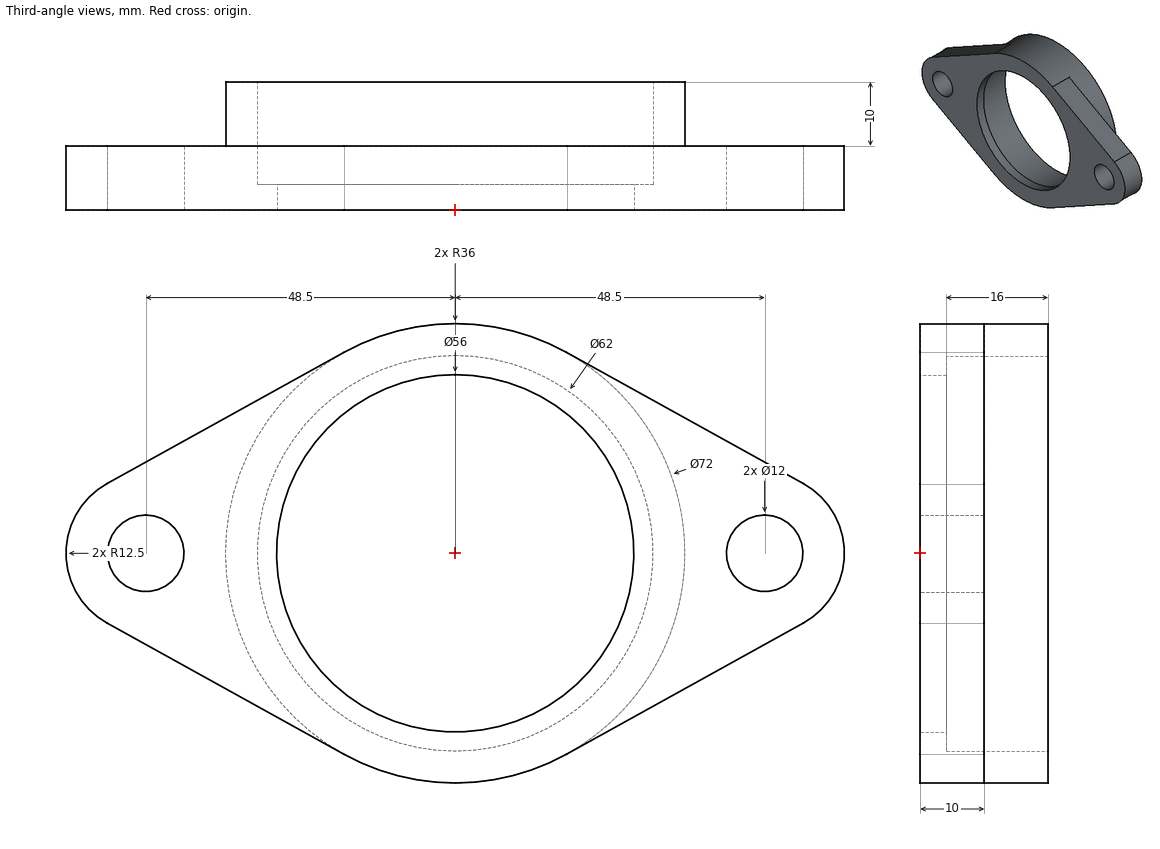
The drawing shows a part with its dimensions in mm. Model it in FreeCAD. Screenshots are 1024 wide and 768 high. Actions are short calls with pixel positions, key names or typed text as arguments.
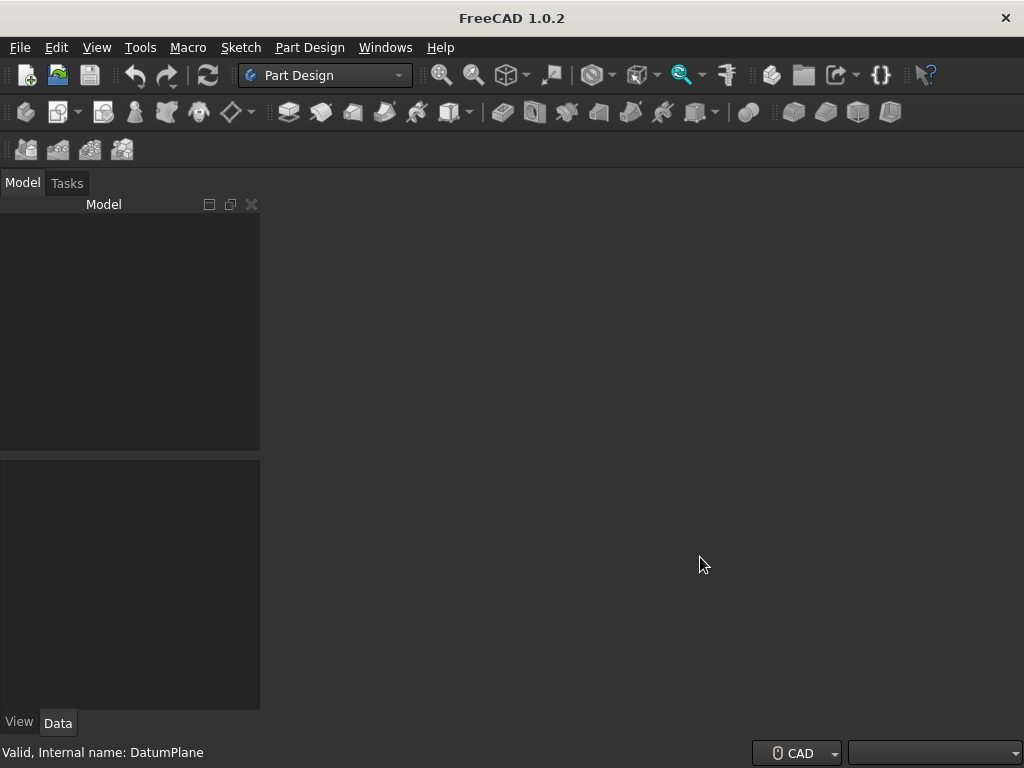
click(26, 76)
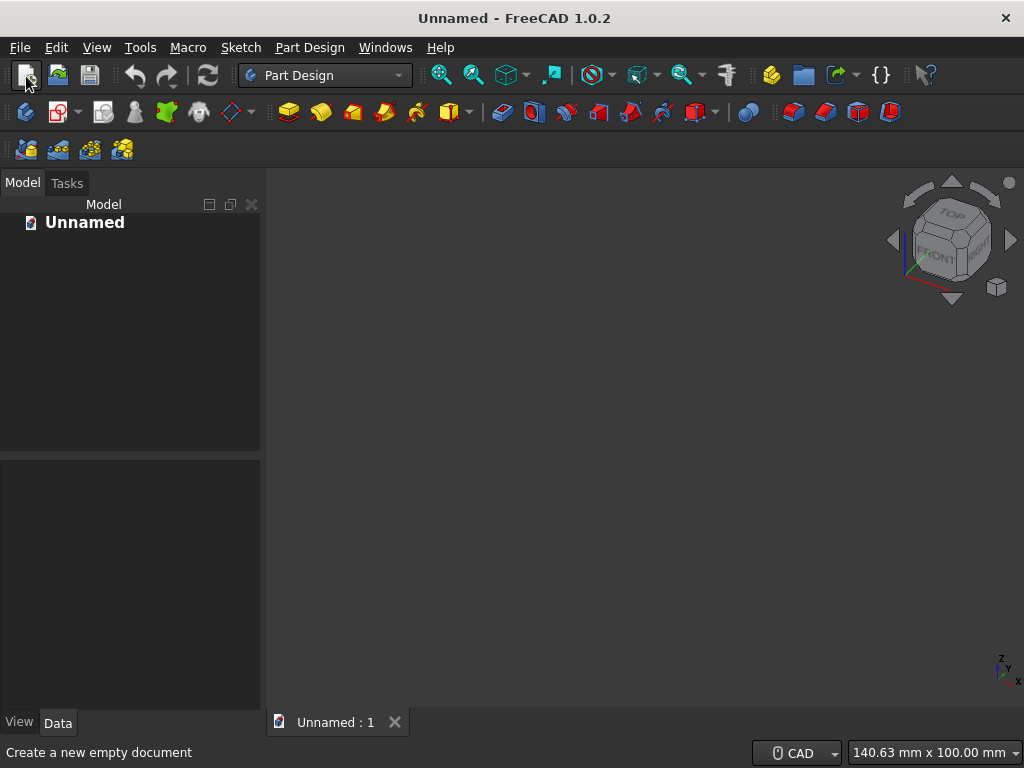
click(58, 112)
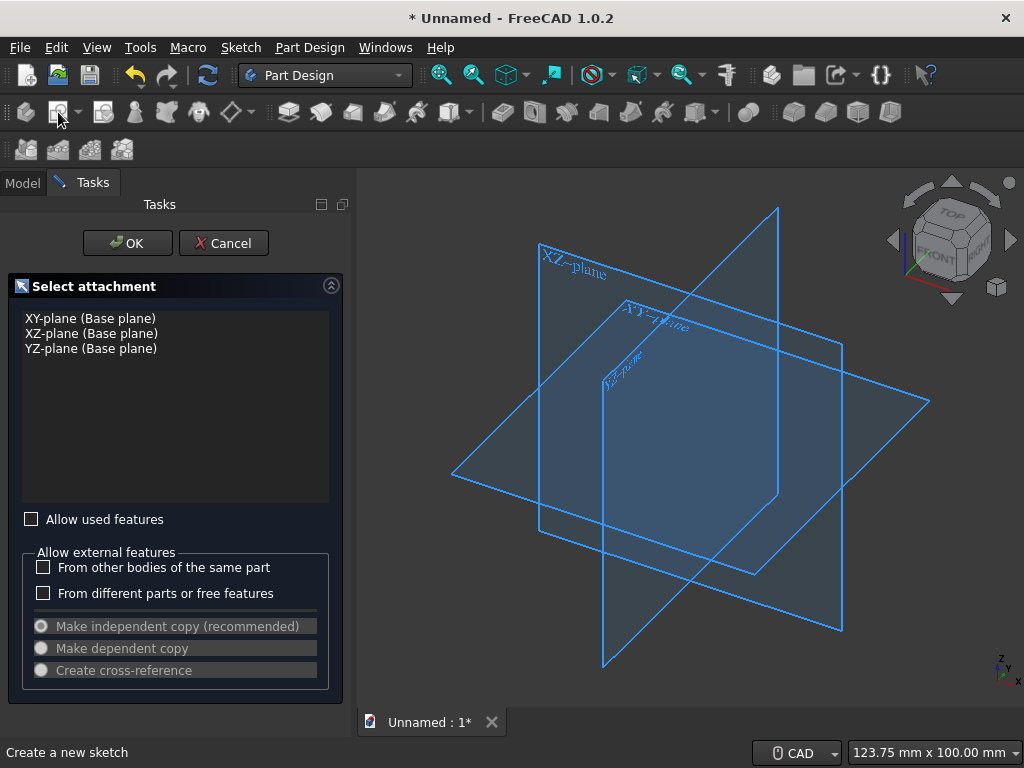
click(82, 334)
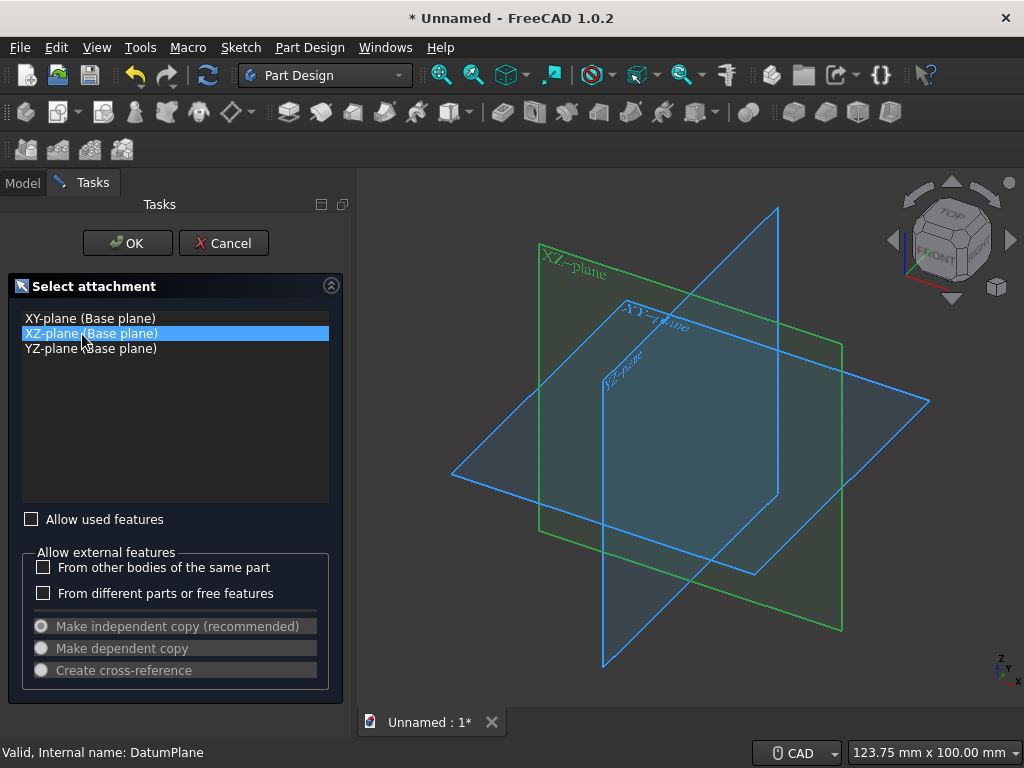
click(128, 243)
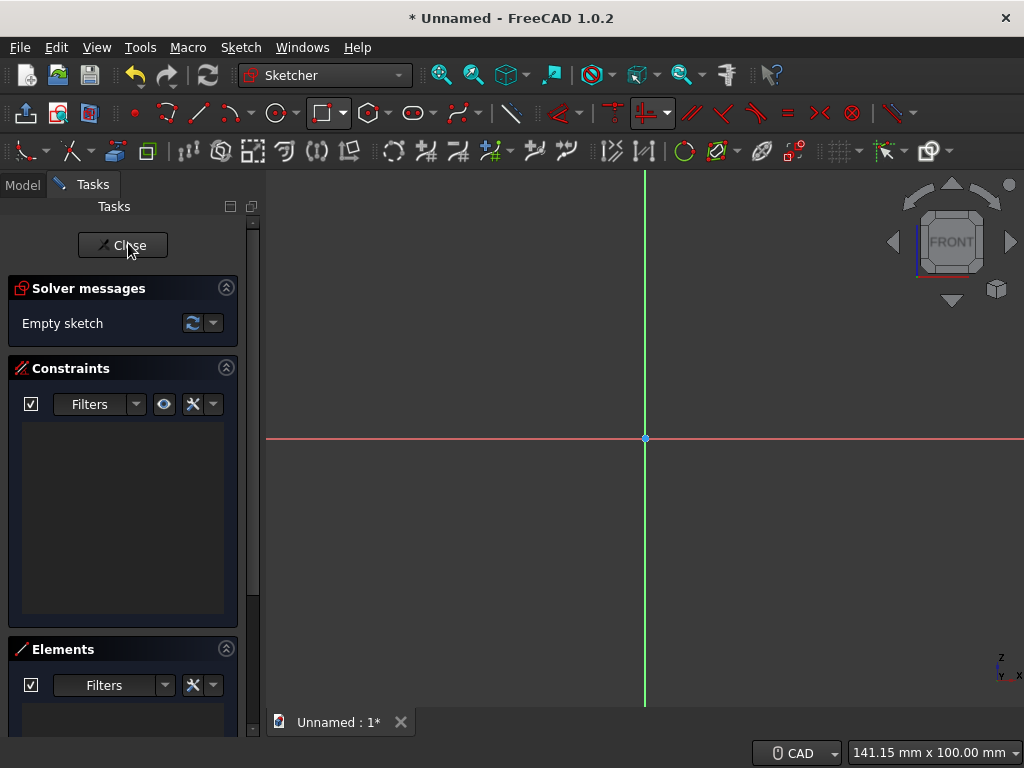
scroll(437, 438, down, 2)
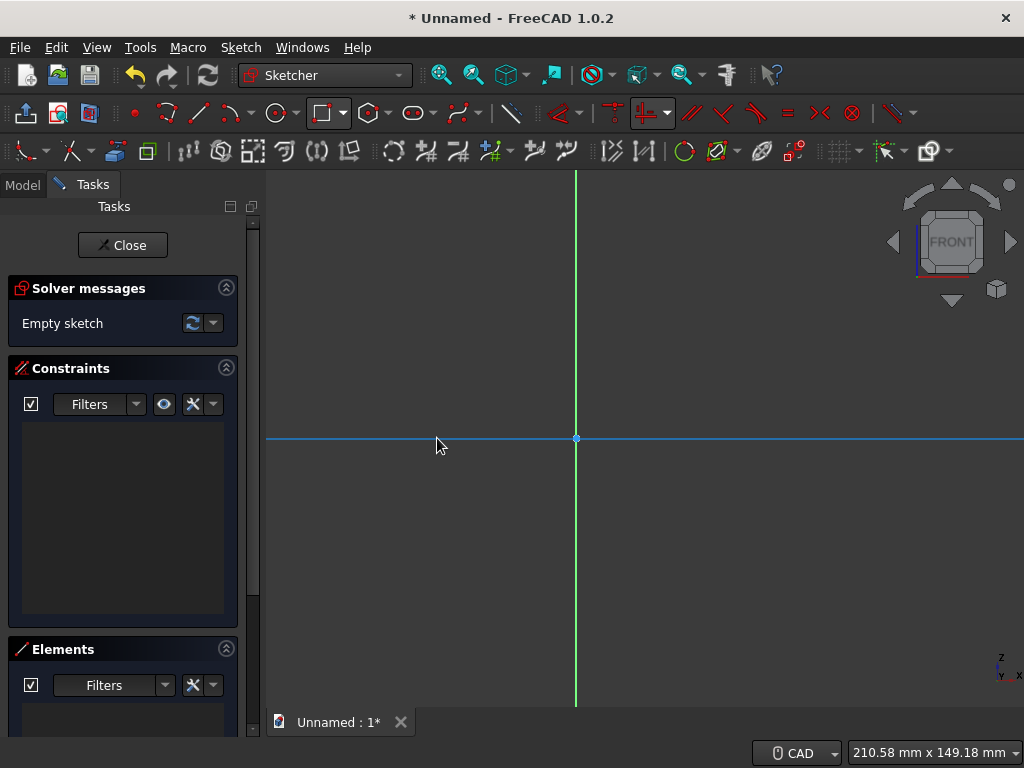
click(200, 114)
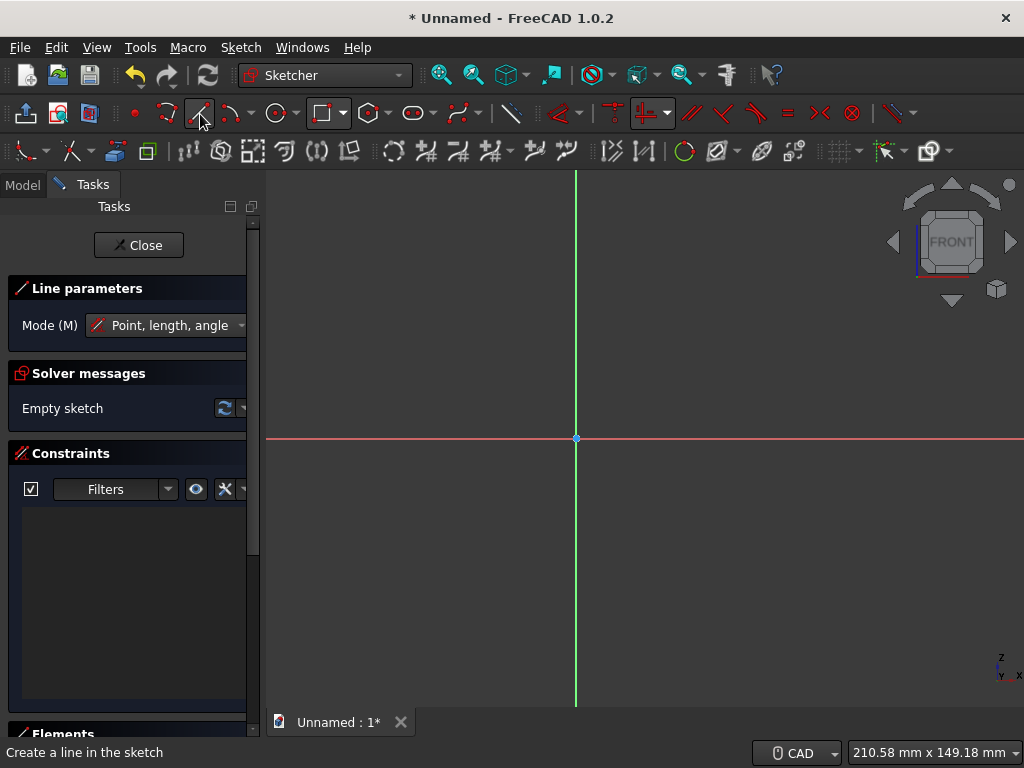
click(514, 552)
click(380, 478)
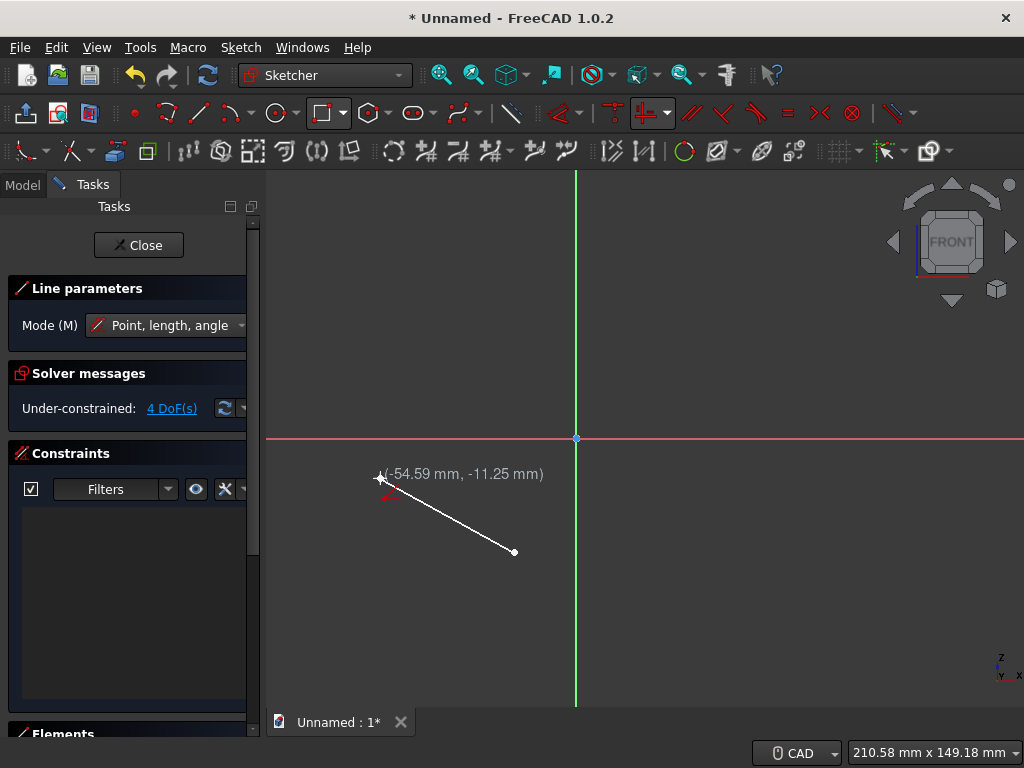
click(380, 399)
click(514, 325)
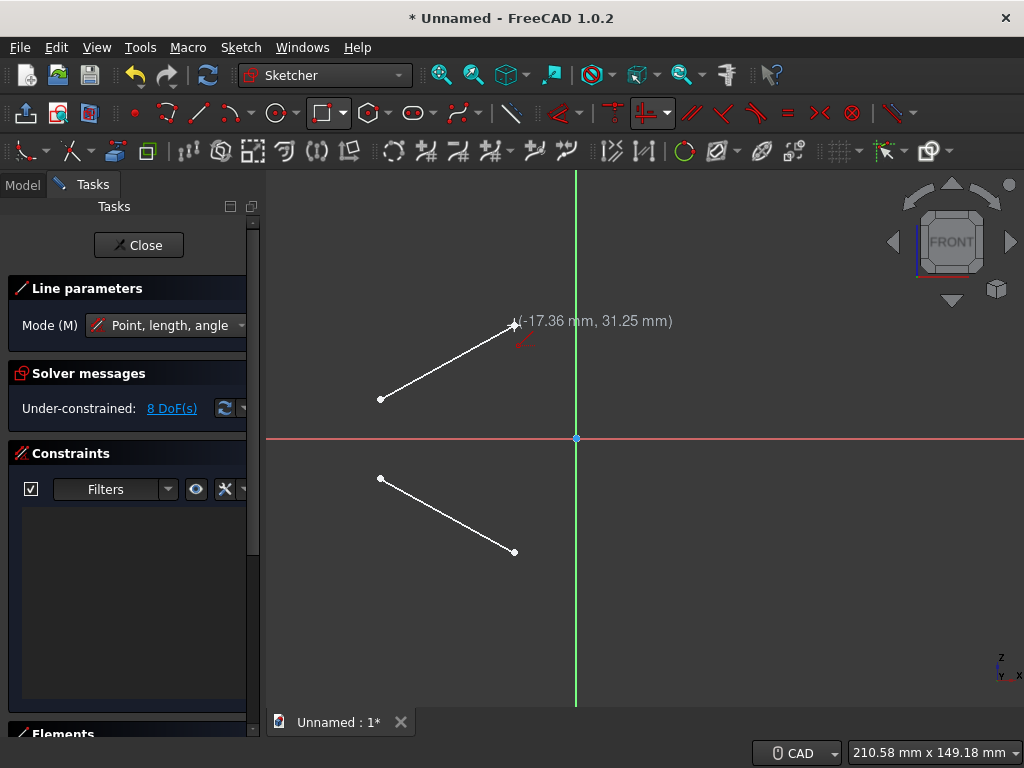
click(639, 325)
click(773, 399)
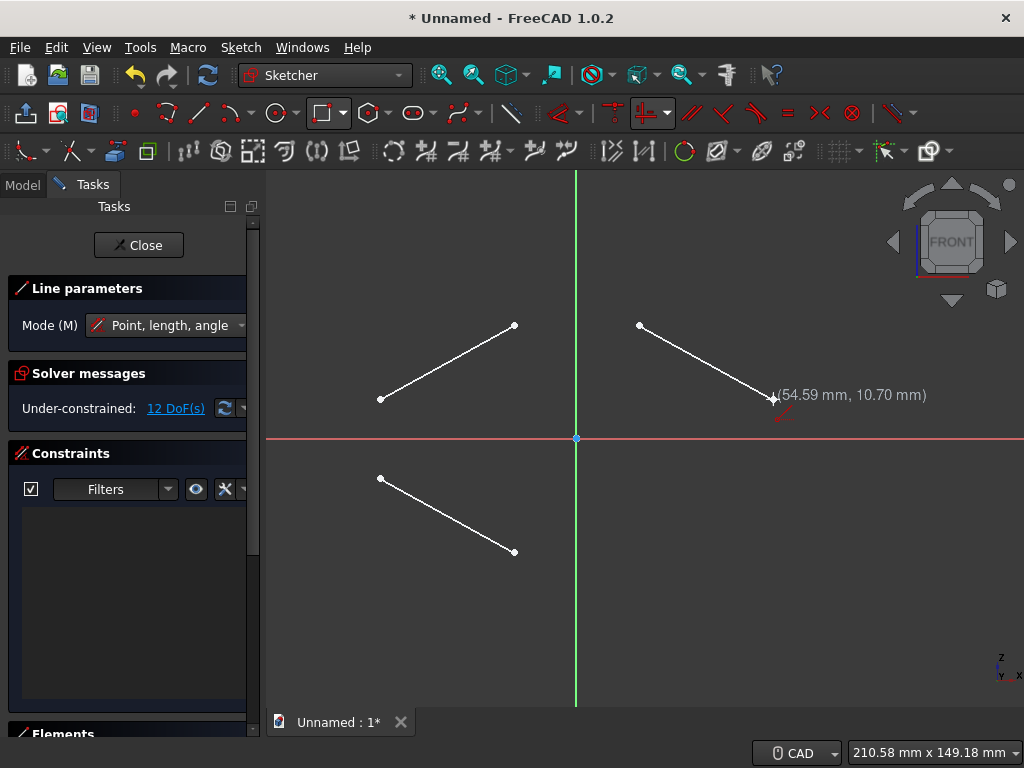
click(773, 478)
click(639, 552)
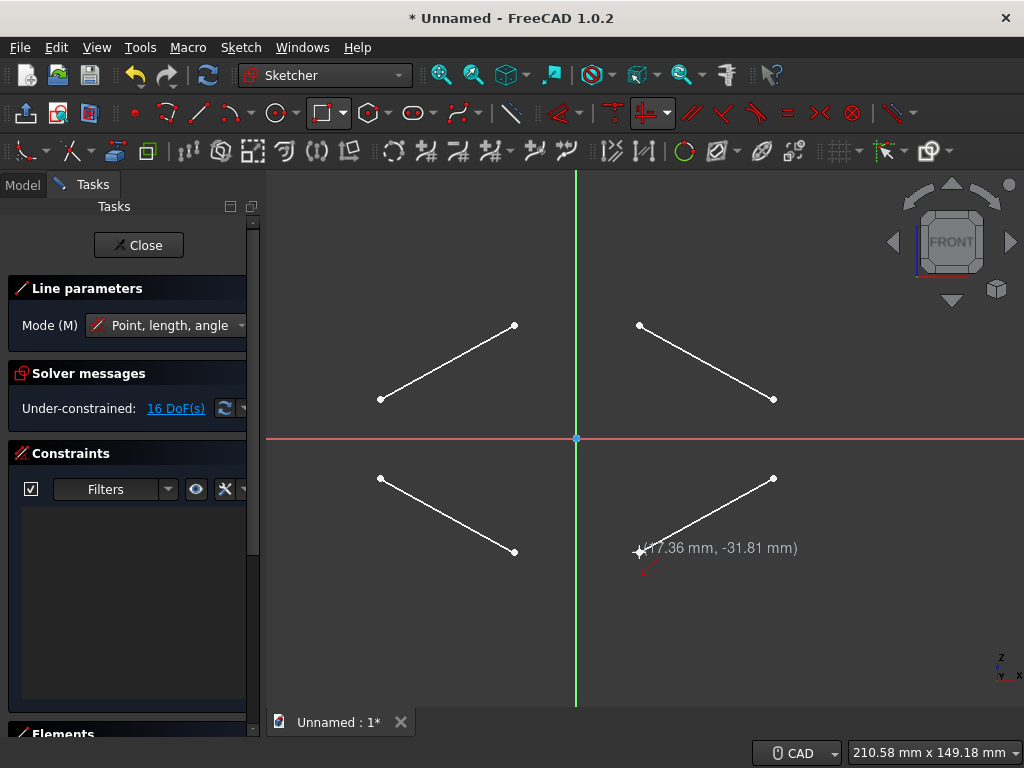
click(254, 114)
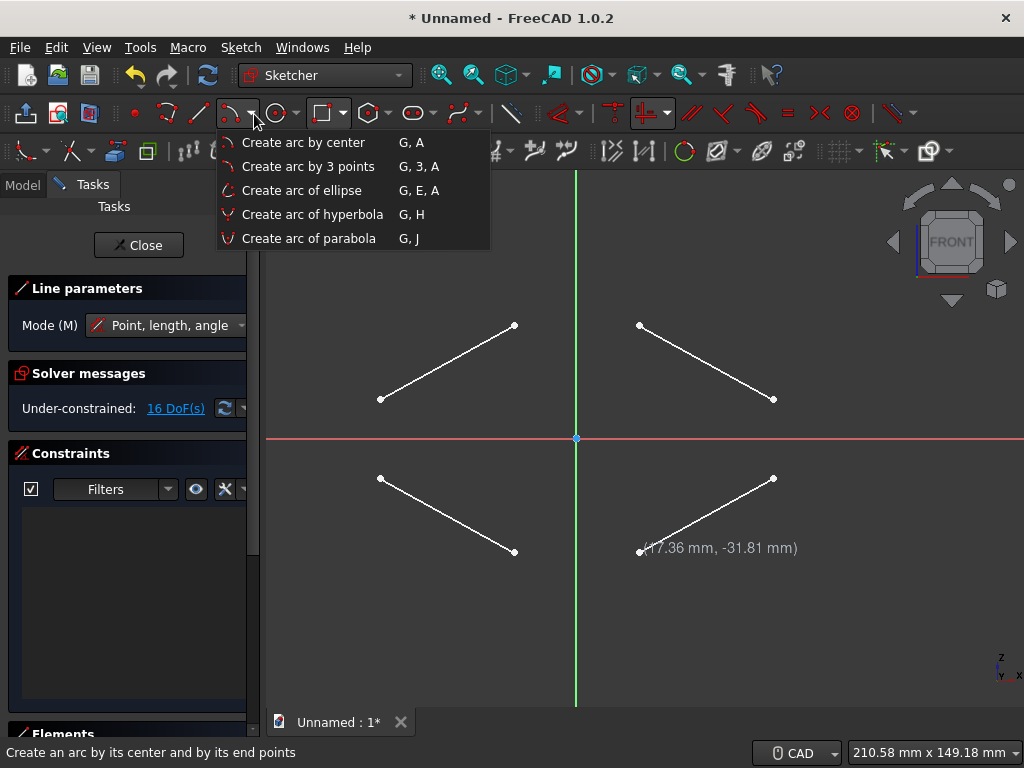
click(354, 166)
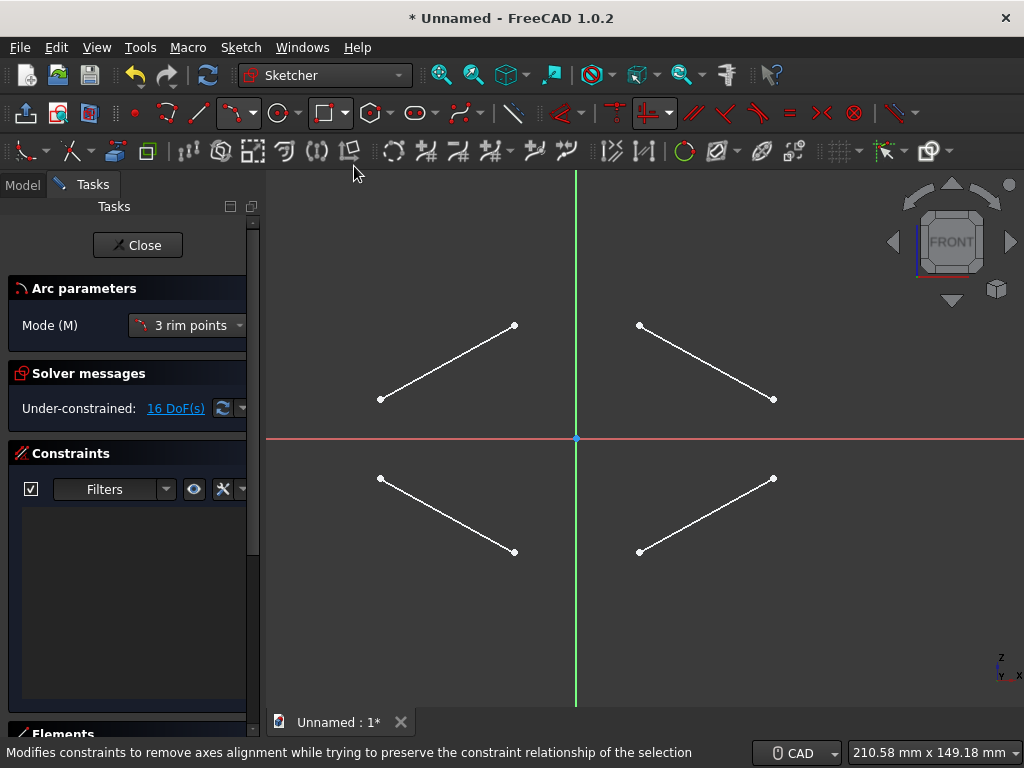
click(380, 479)
click(380, 400)
click(361, 420)